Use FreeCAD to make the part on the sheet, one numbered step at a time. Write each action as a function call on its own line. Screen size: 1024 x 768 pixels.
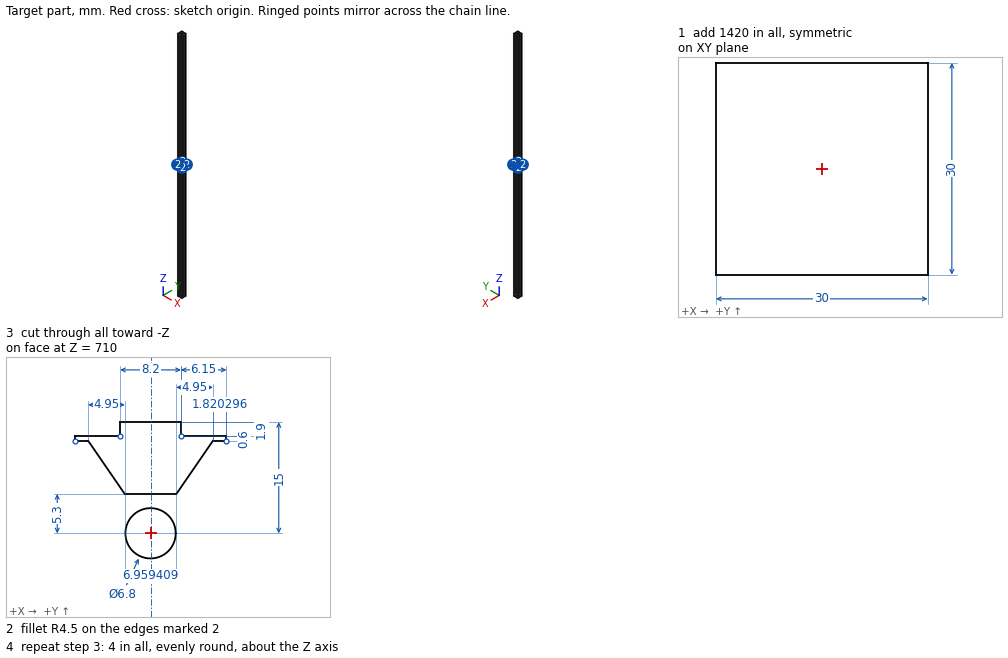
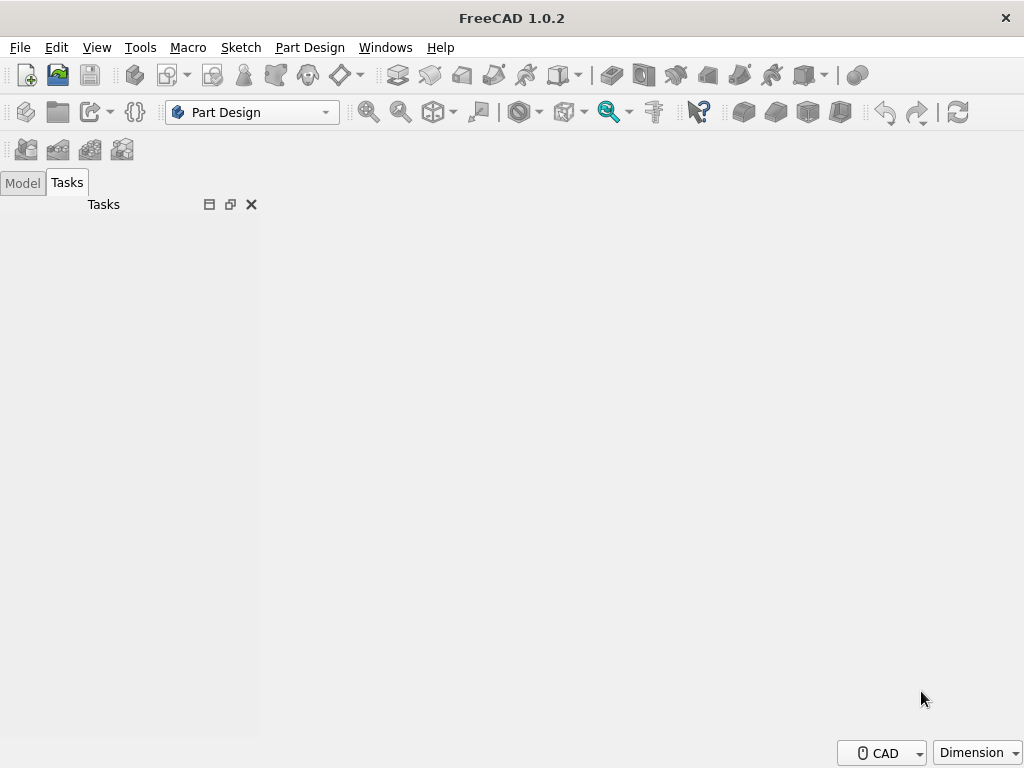
click(26, 76)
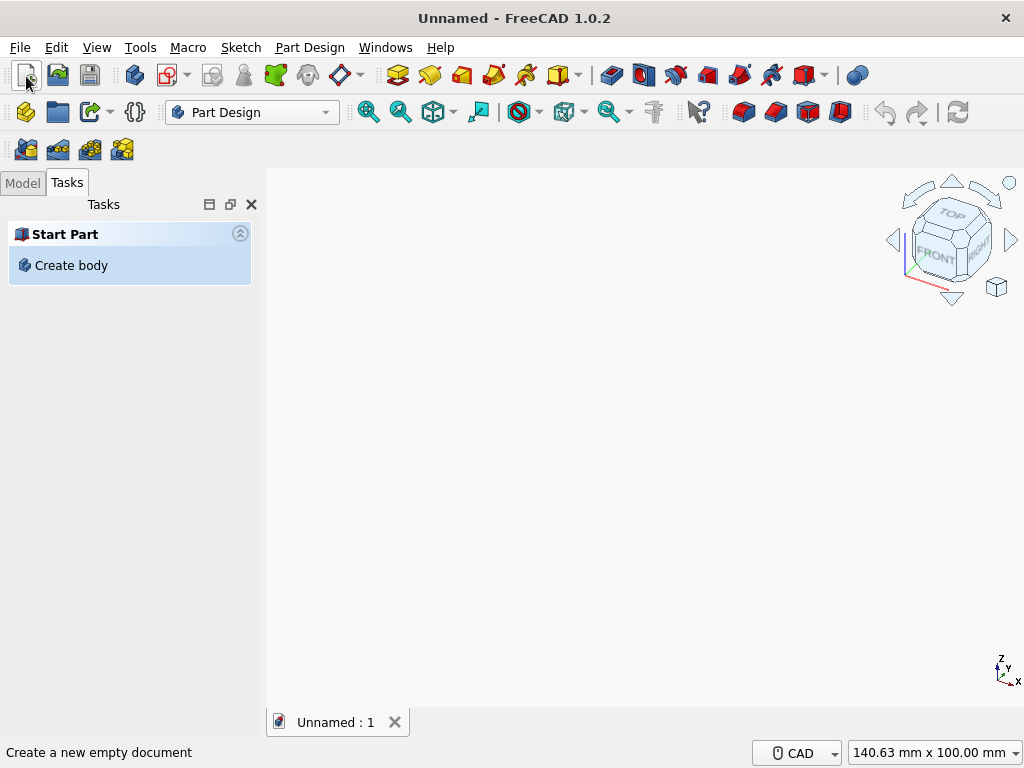
click(168, 76)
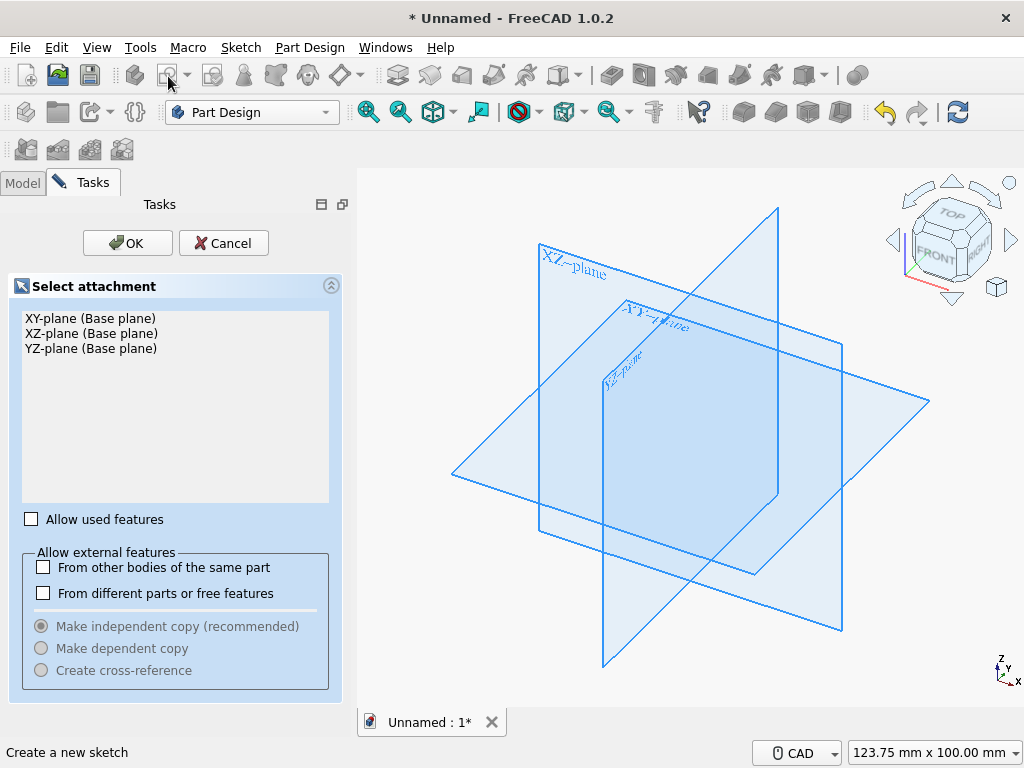
click(82, 318)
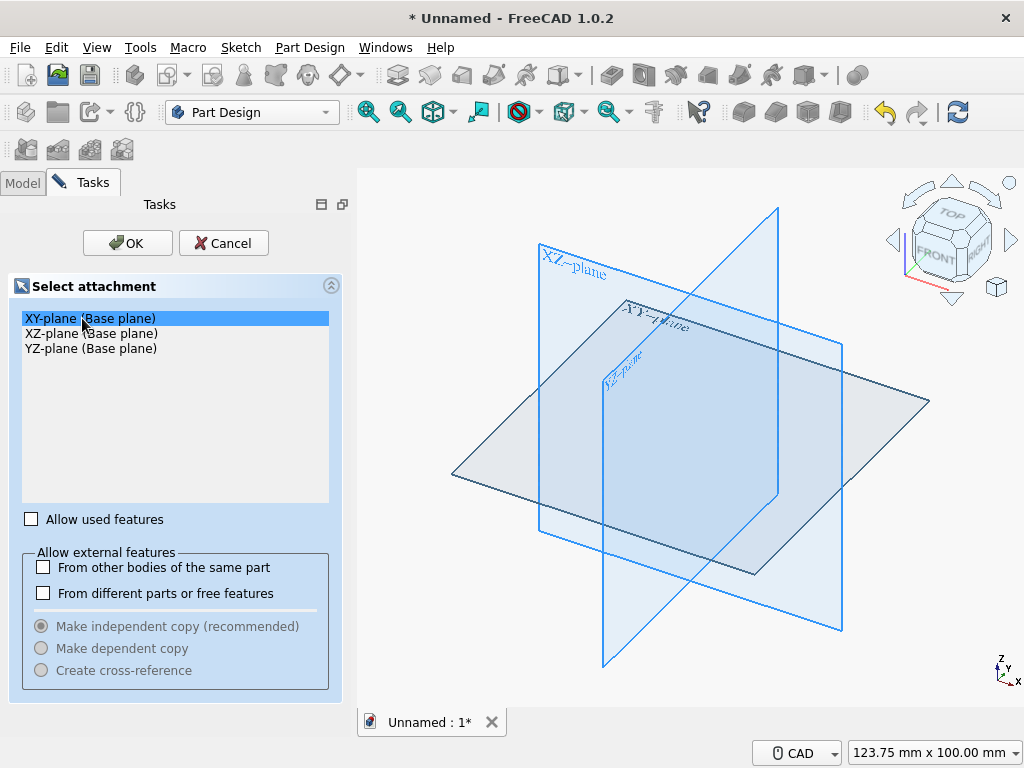
click(128, 243)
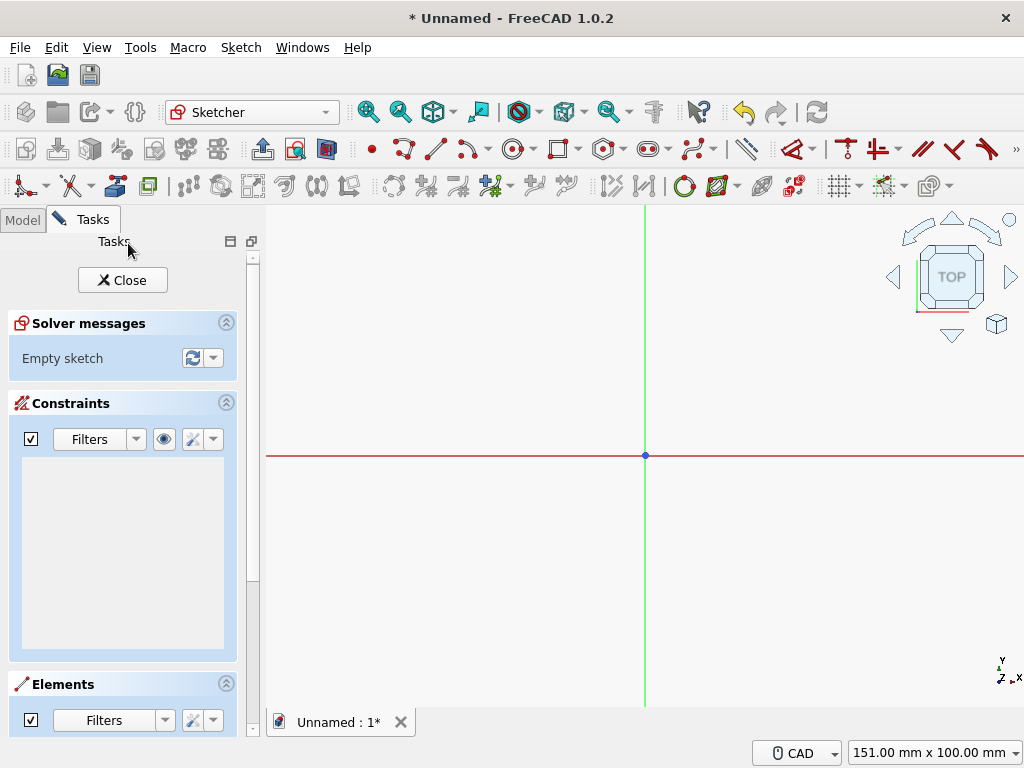
scroll(701, 456, up, 4)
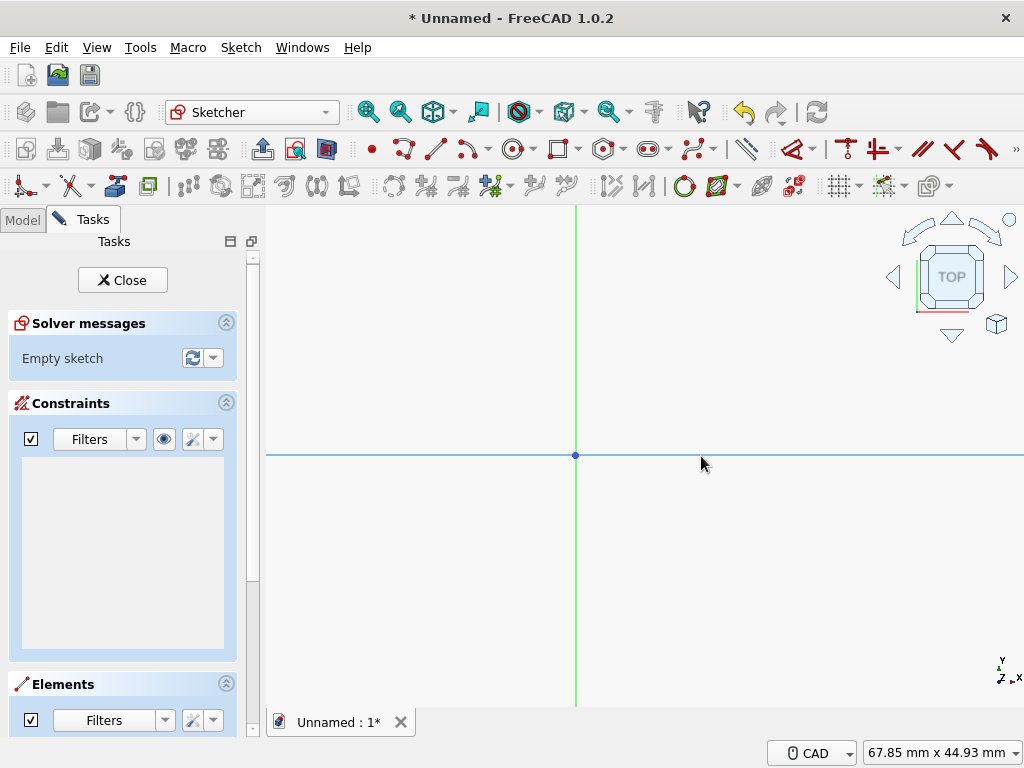
key(g)
key(v)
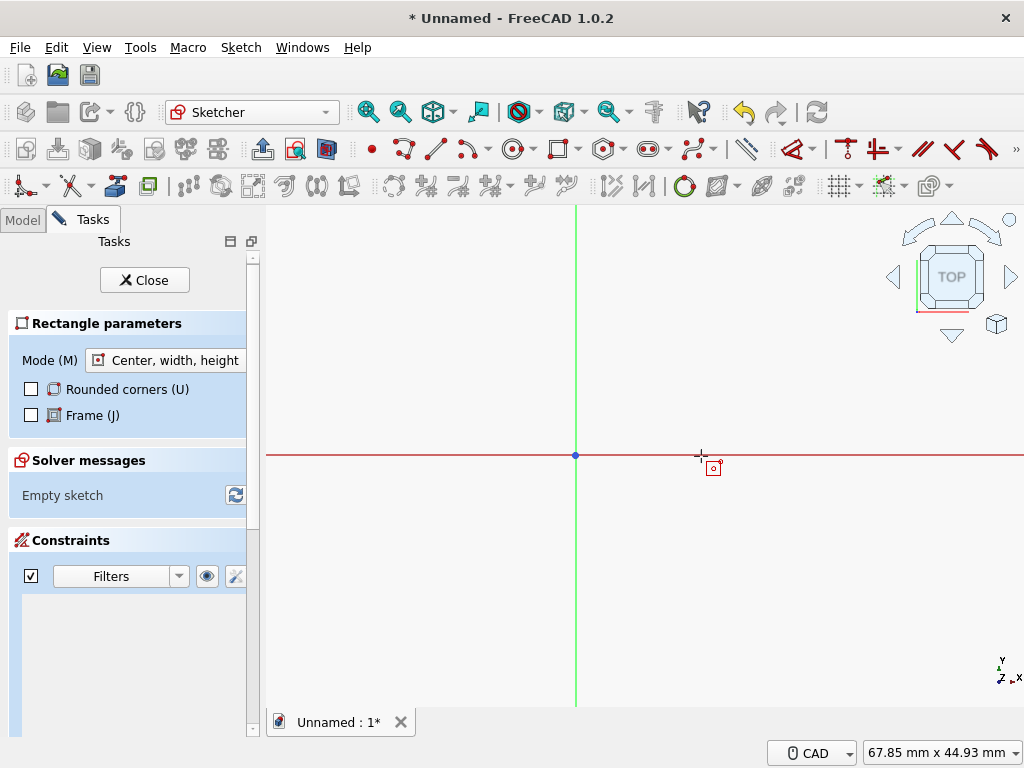
click(576, 455)
click(743, 288)
key(Escape)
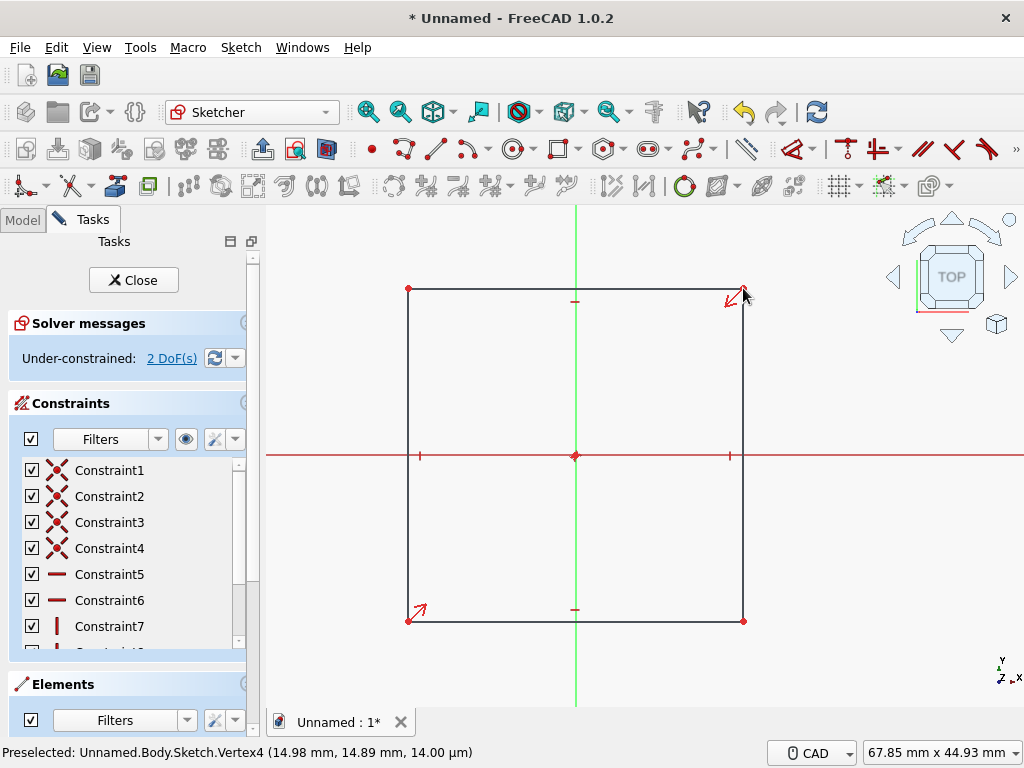
key(d)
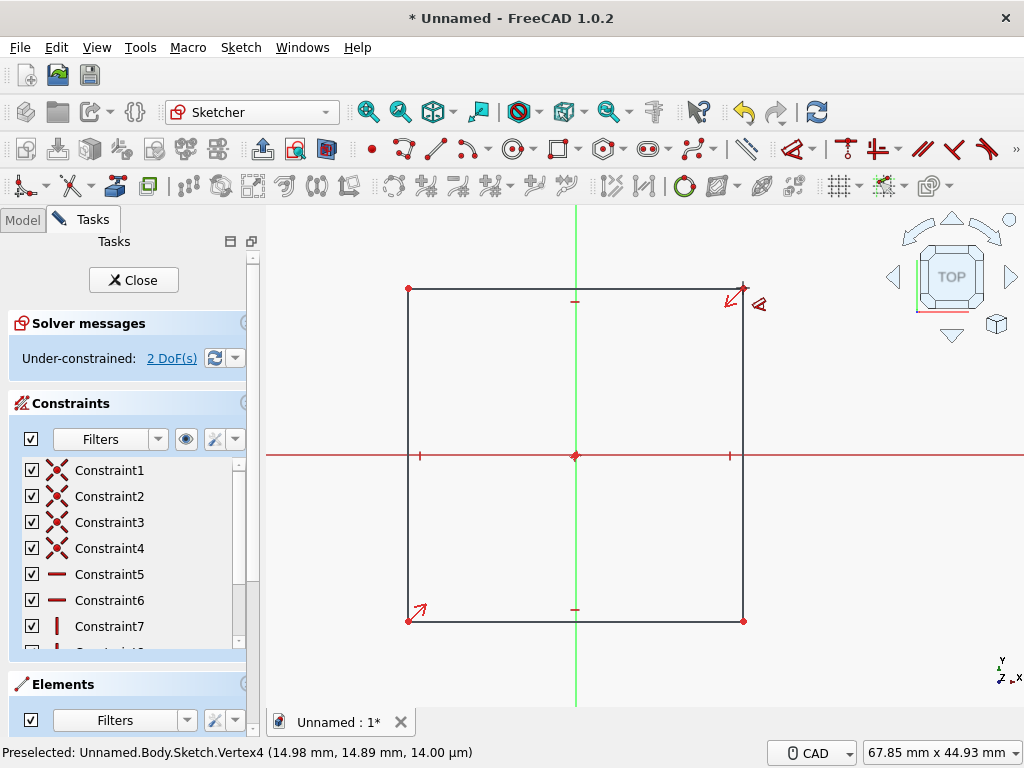
click(509, 622)
click(499, 656)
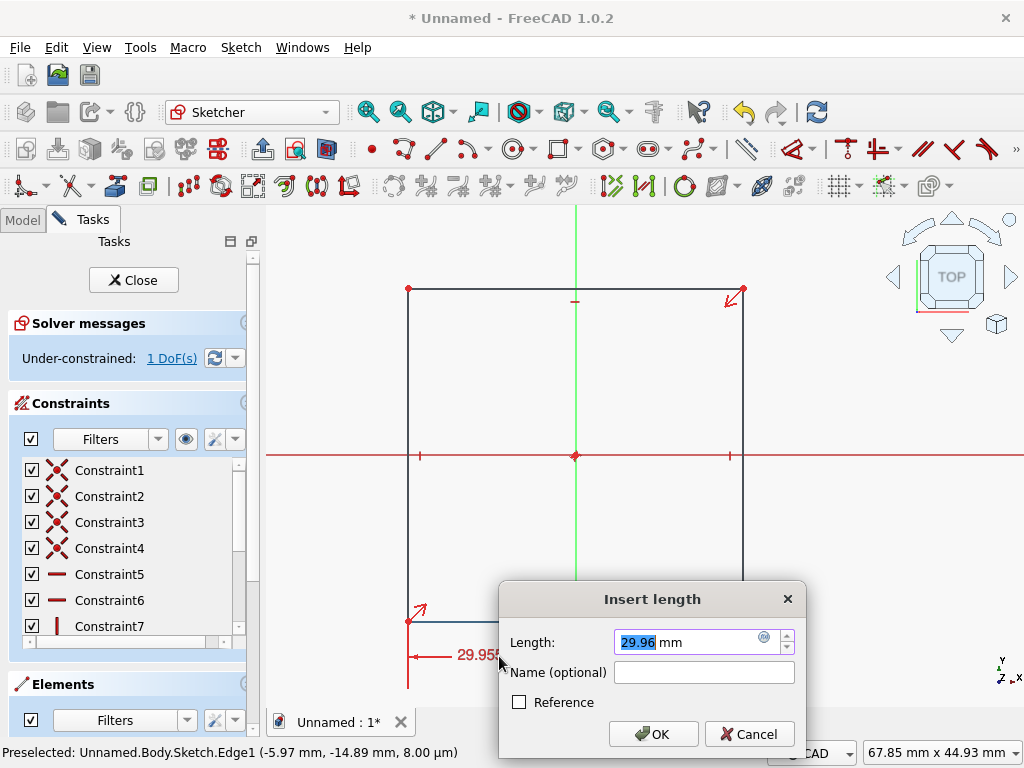
text(30)
key(Return)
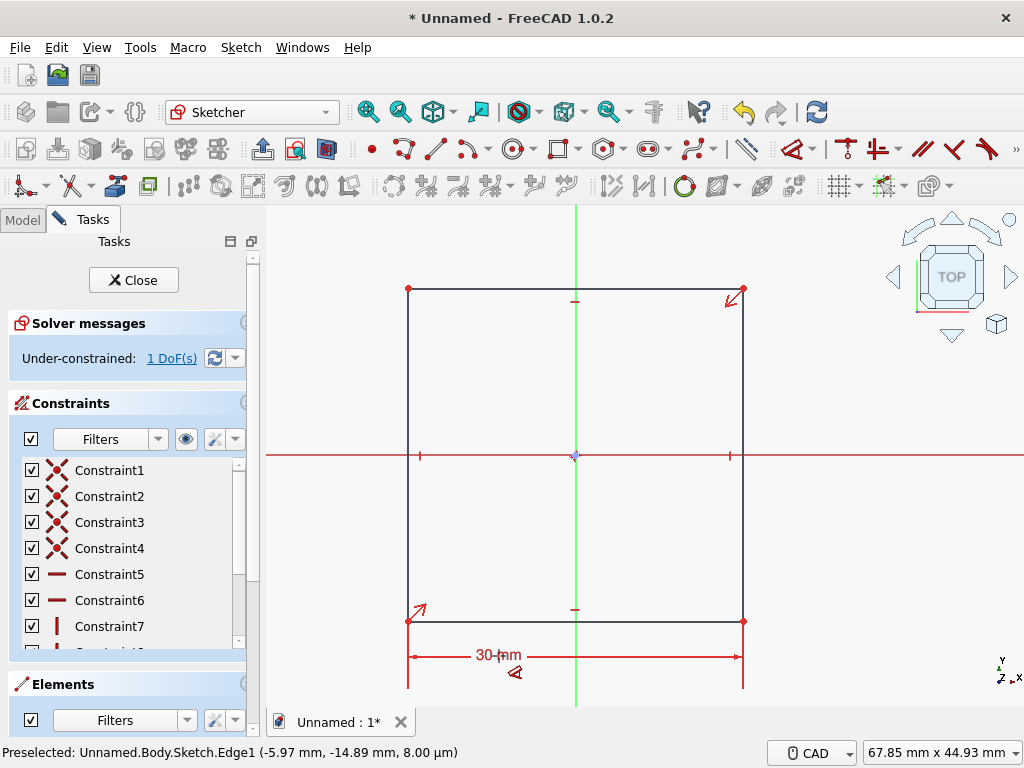
click(743, 522)
click(777, 379)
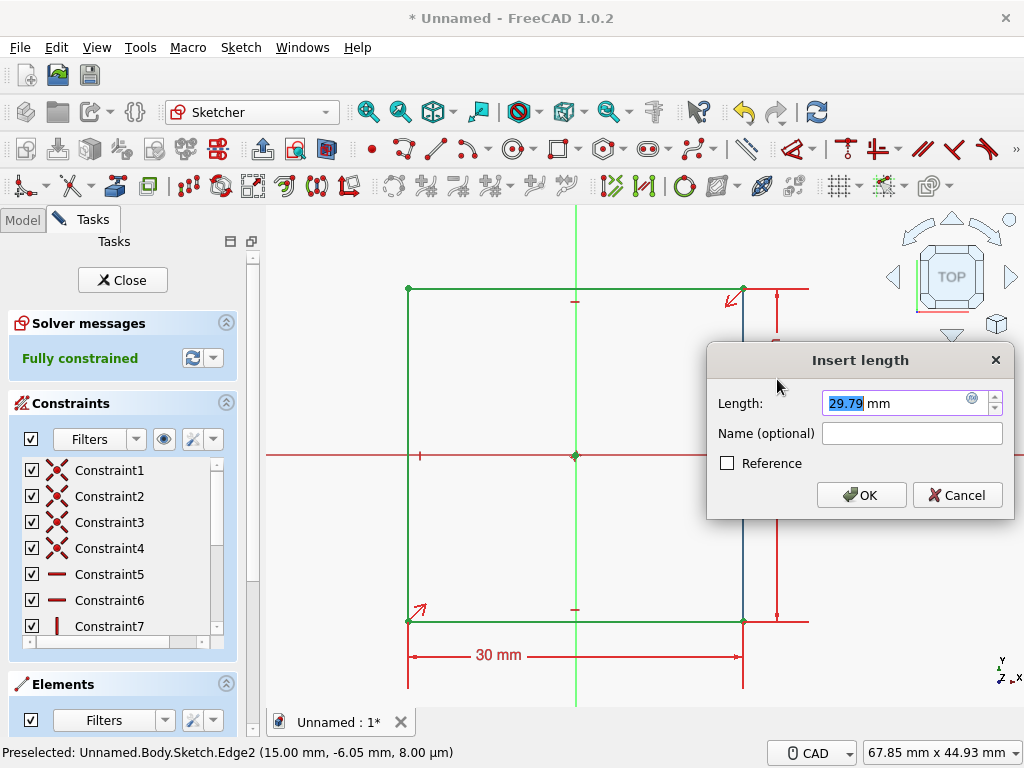
text(30)
key(Return)
key(Escape)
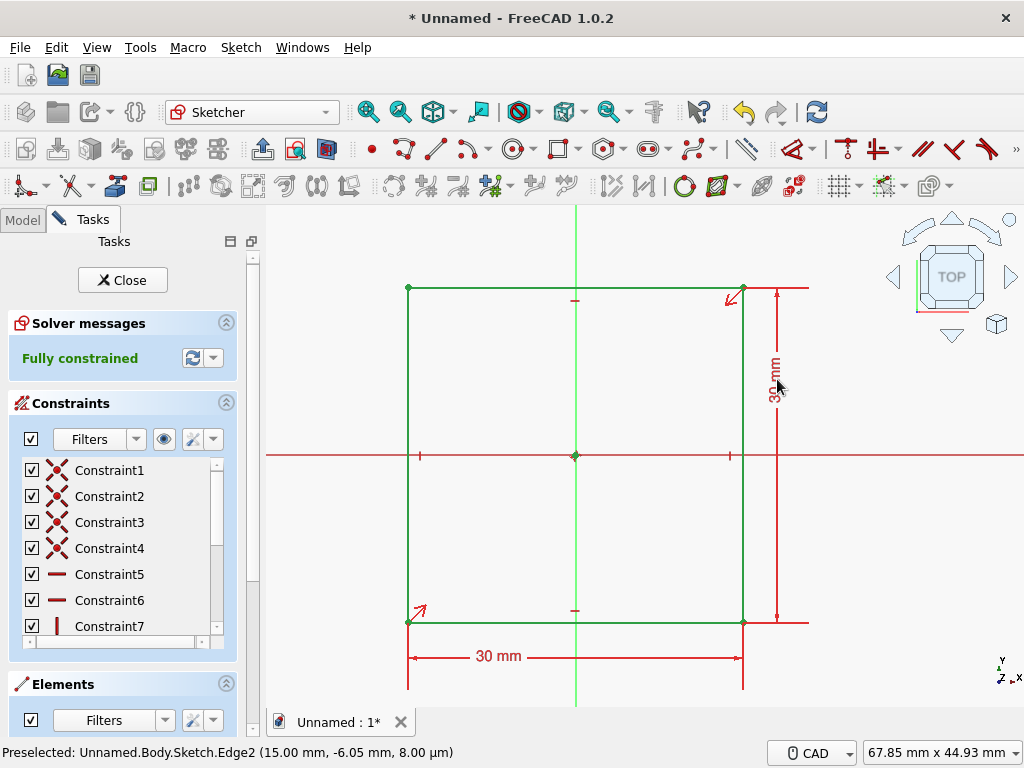
click(123, 280)